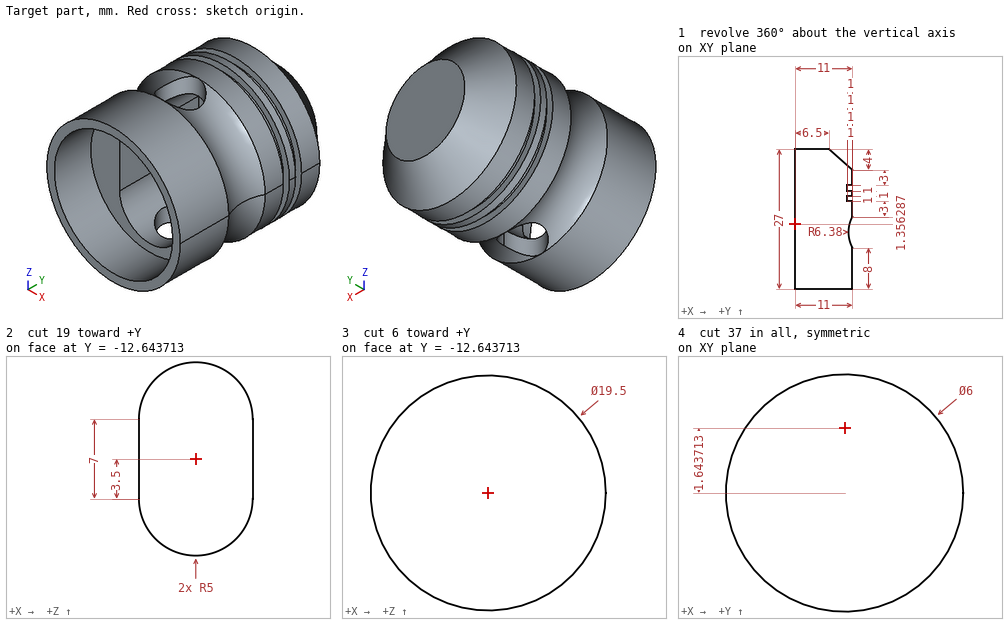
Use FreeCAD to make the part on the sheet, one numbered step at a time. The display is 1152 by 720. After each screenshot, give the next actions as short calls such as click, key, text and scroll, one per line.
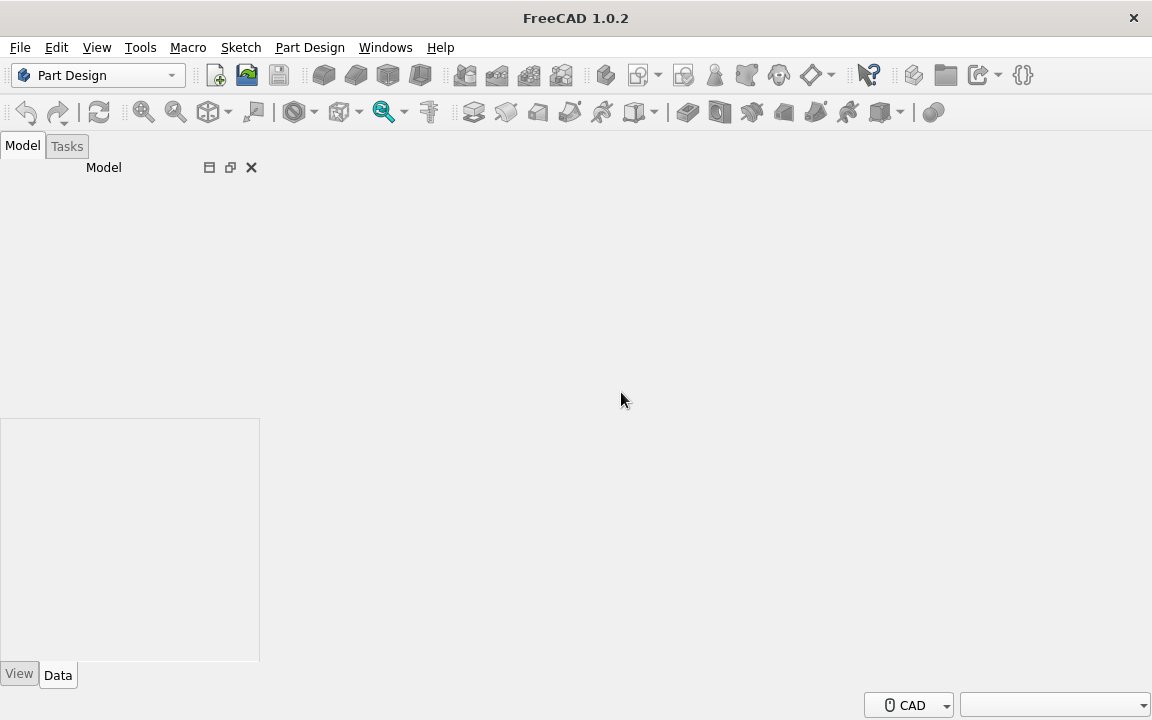
key(ctrl+n)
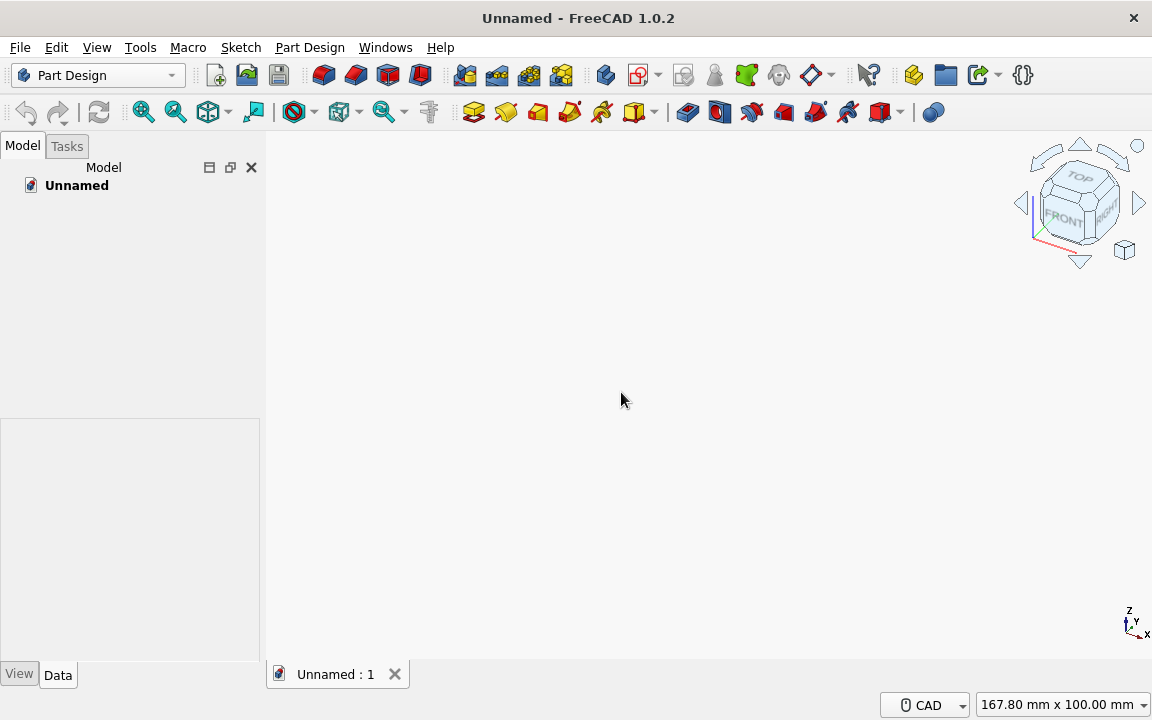
click(638, 76)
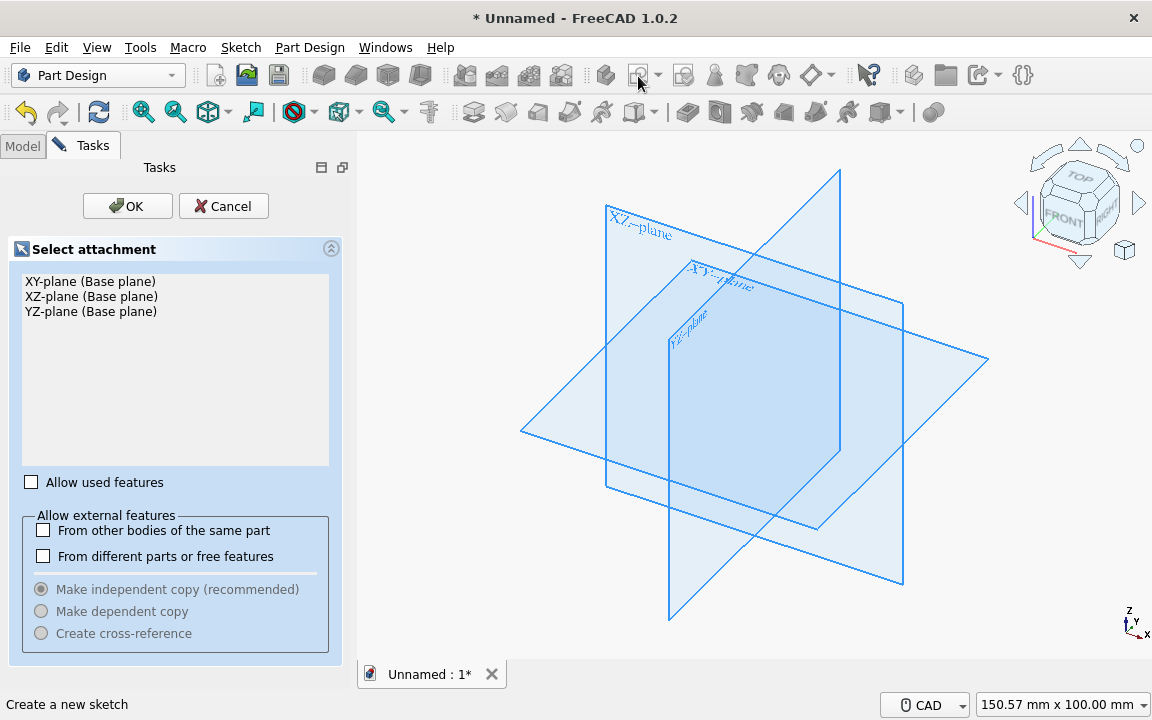
click(82, 282)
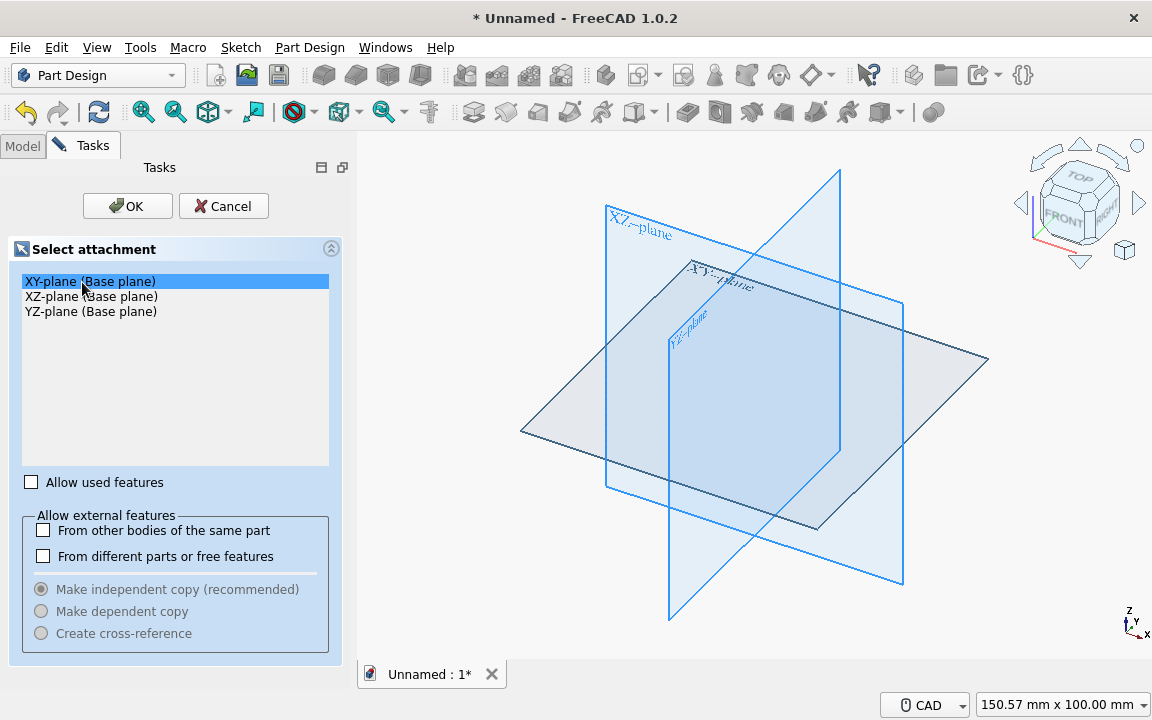
click(128, 206)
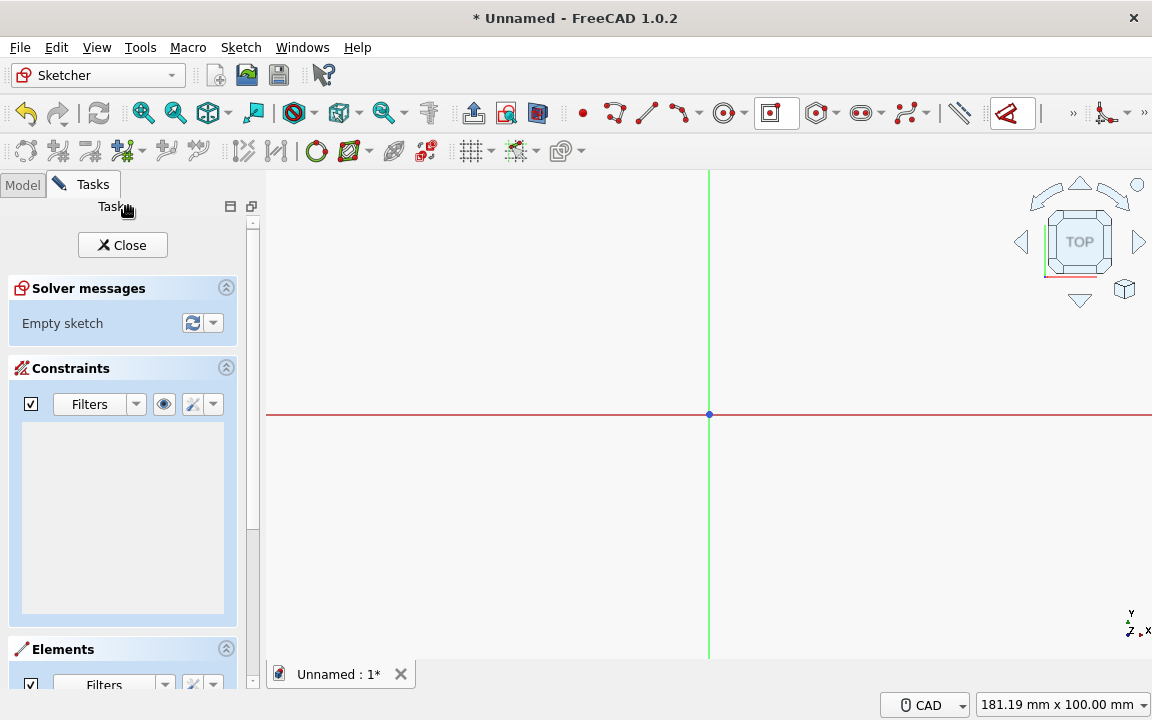
scroll(814, 407, up, 4)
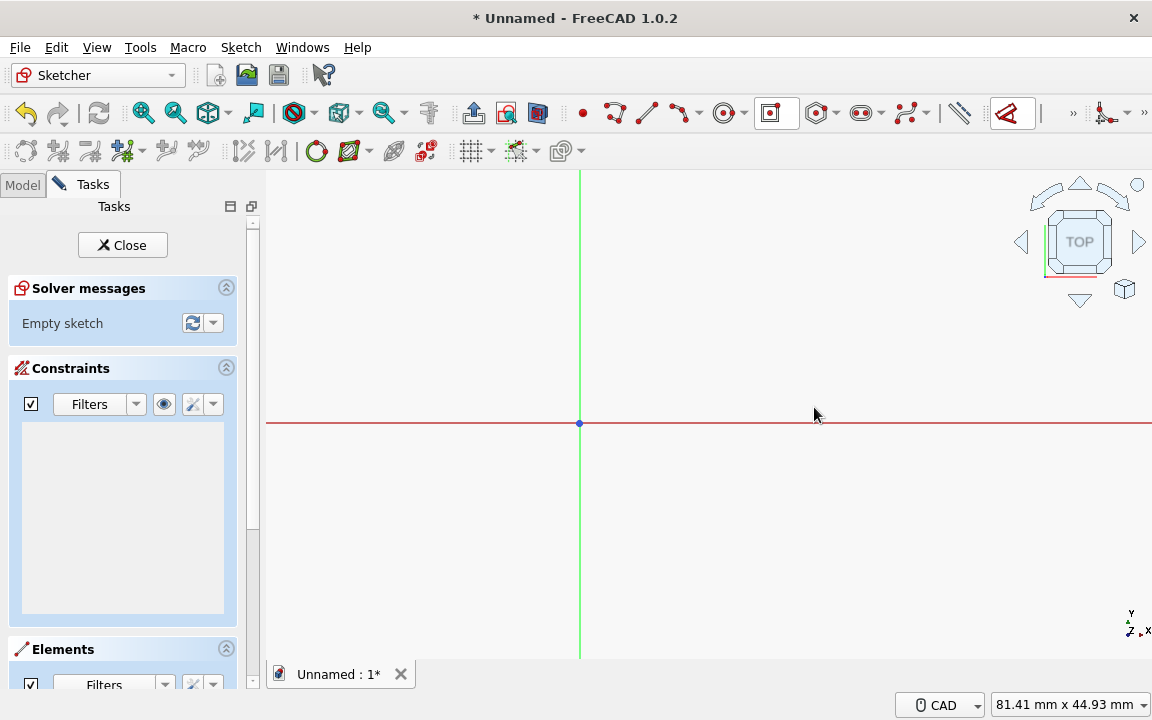
click(616, 114)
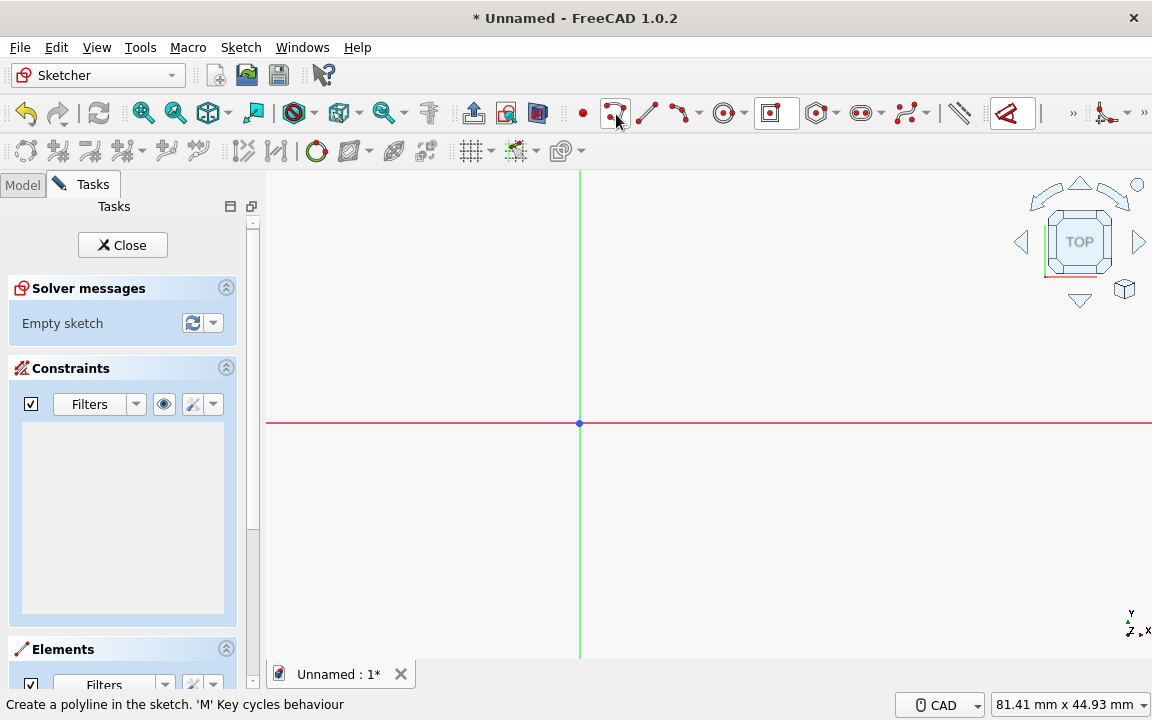
click(699, 408)
click(699, 376)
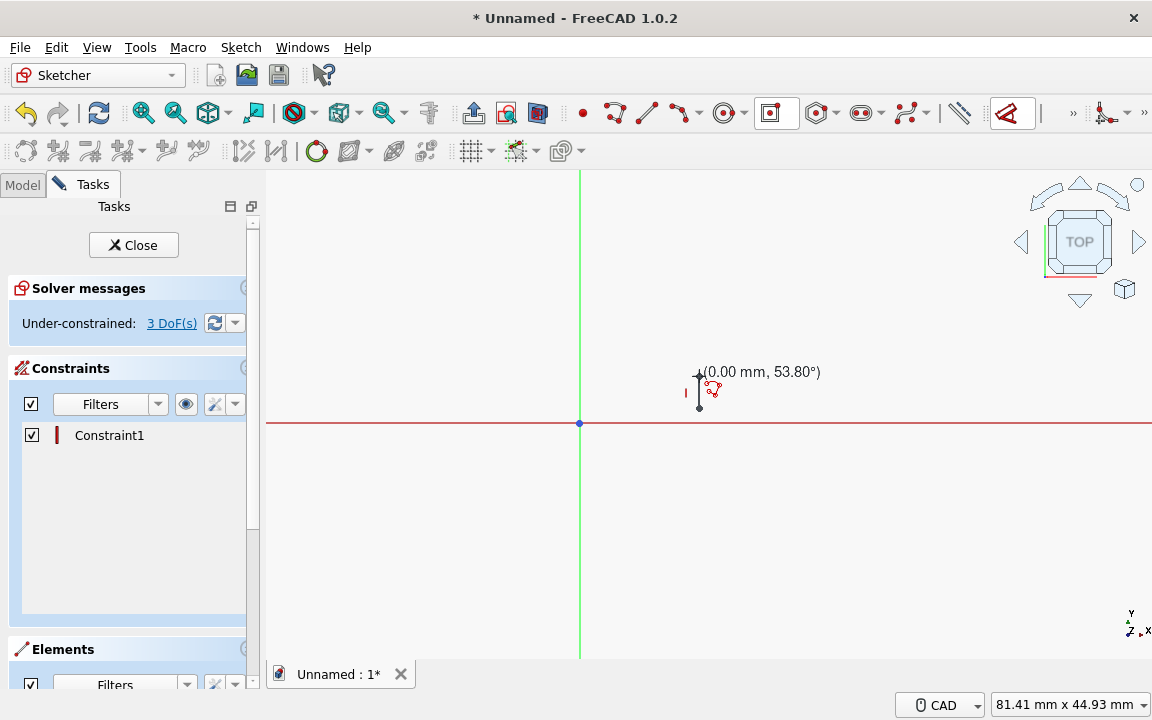
scroll(688, 376, up, 2)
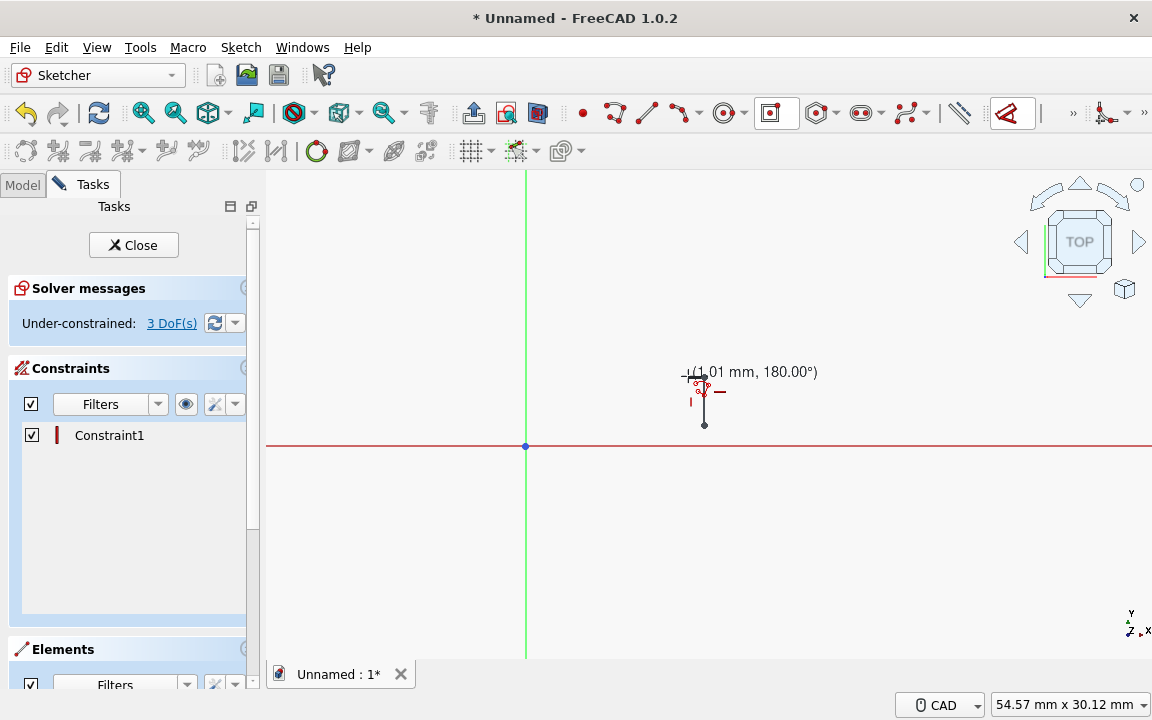
click(688, 376)
click(688, 359)
click(705, 359)
click(705, 343)
click(688, 343)
click(688, 327)
click(705, 327)
click(705, 278)
click(632, 213)
click(526, 213)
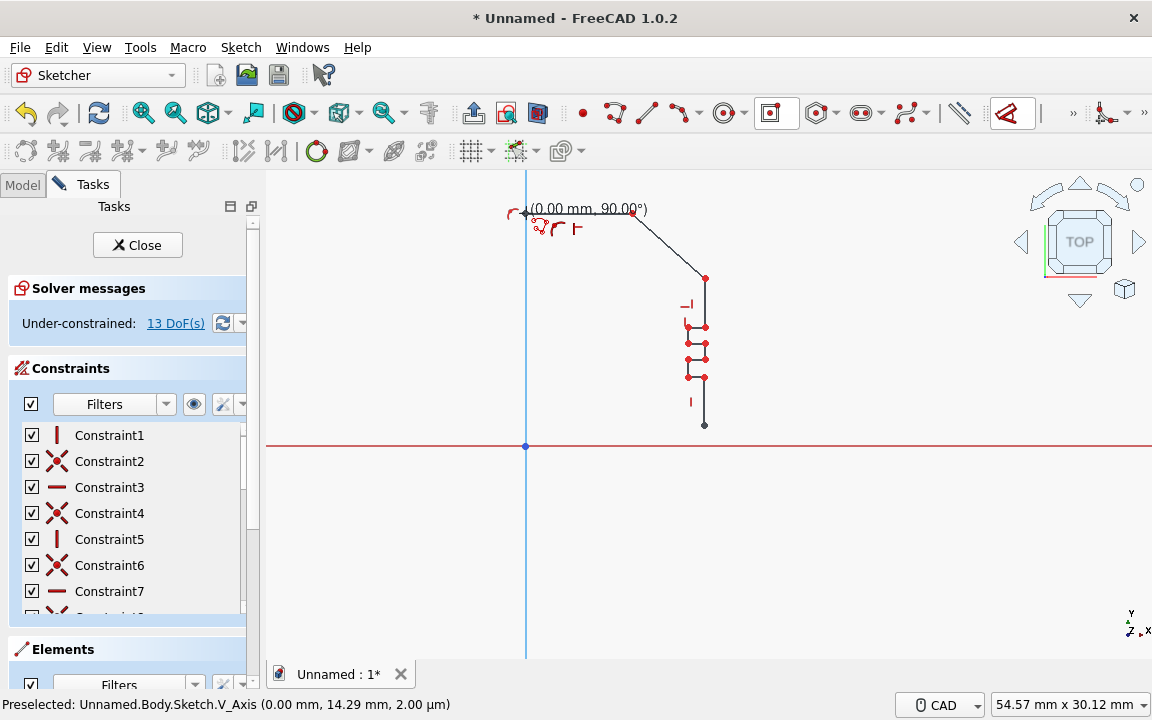
scroll(692, 379, down, 2)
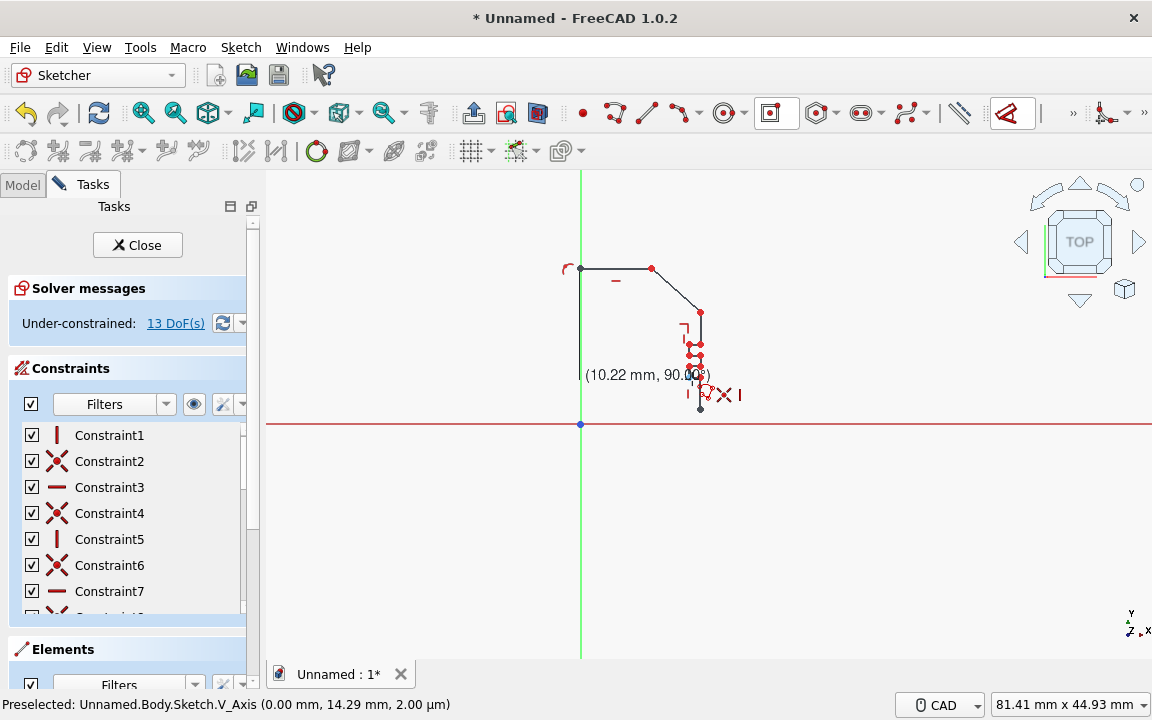
click(590, 562)
click(701, 562)
click(701, 475)
right_click(701, 475)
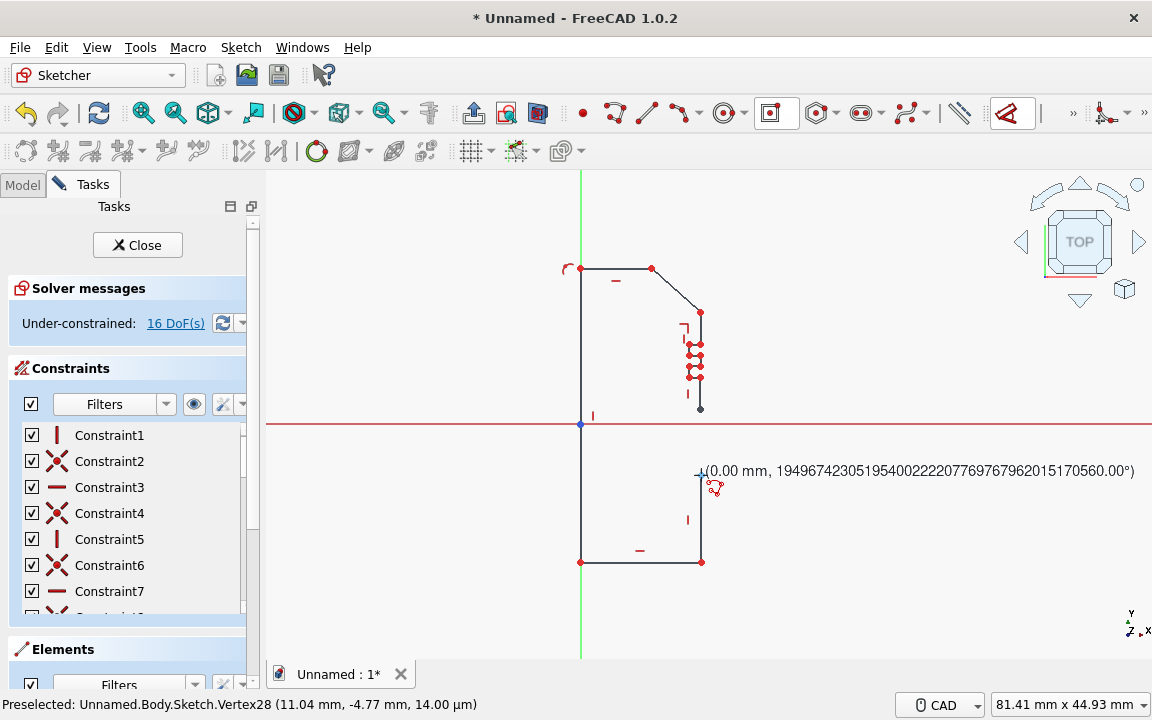
click(680, 114)